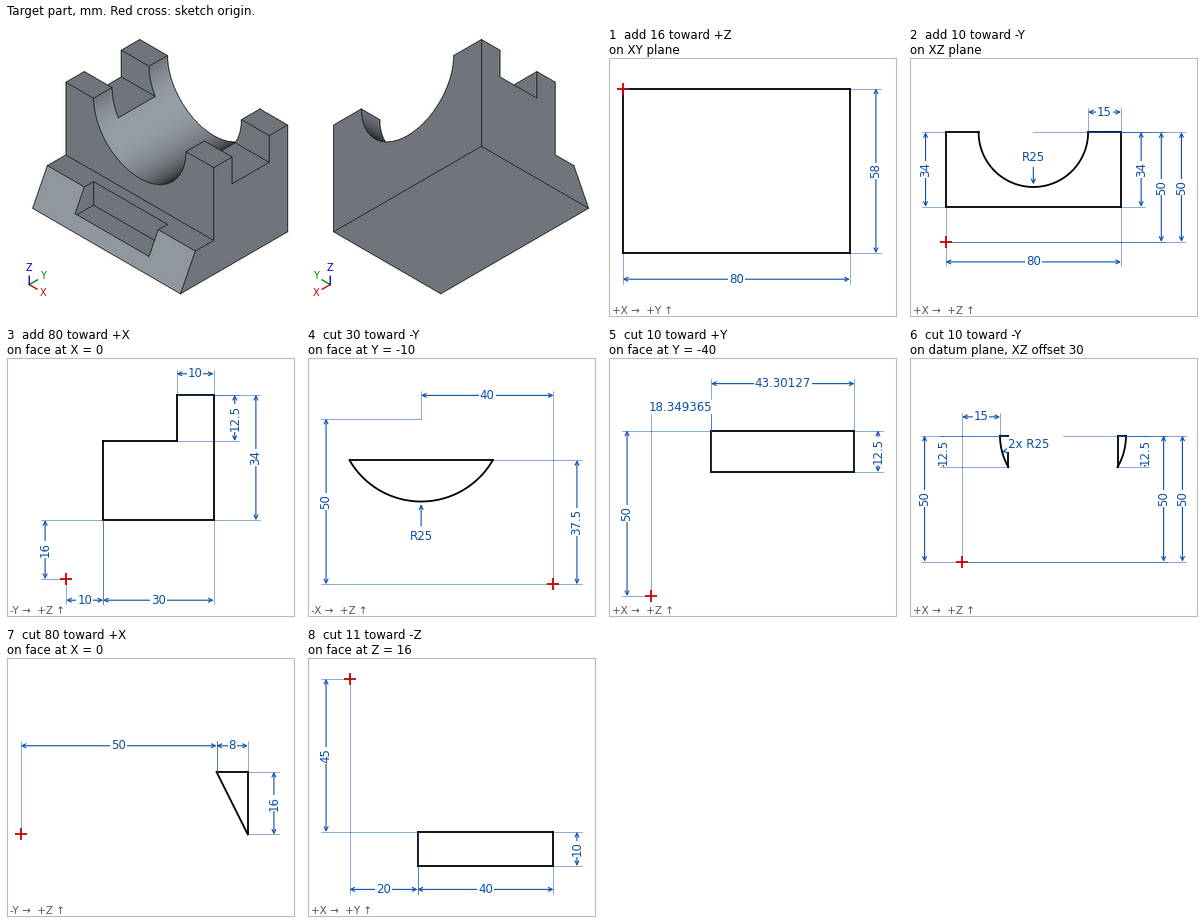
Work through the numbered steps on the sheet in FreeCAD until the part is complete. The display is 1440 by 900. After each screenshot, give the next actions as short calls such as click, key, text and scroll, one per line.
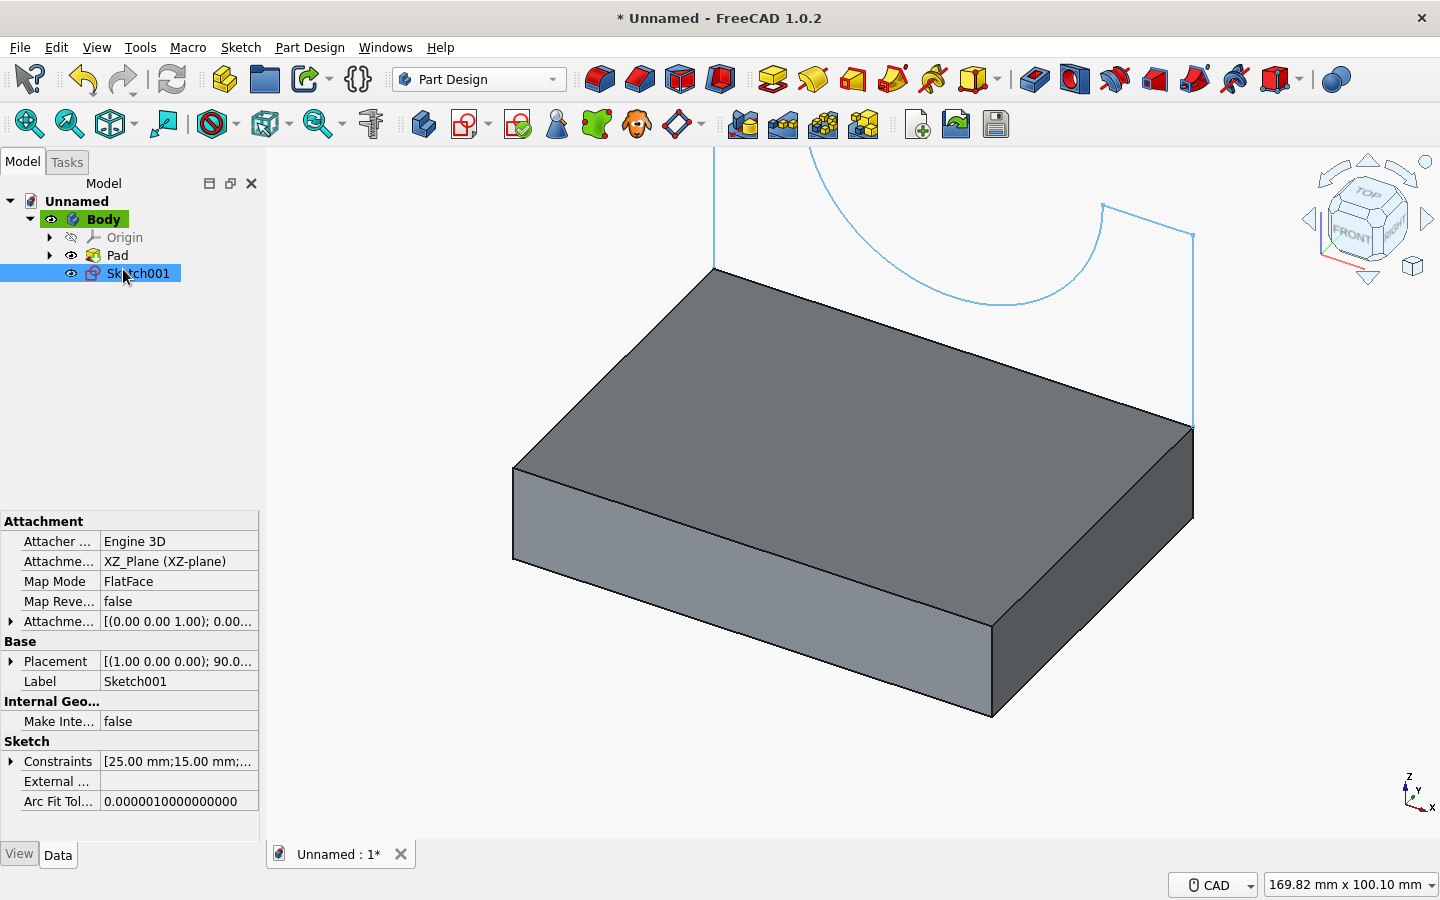
click(774, 80)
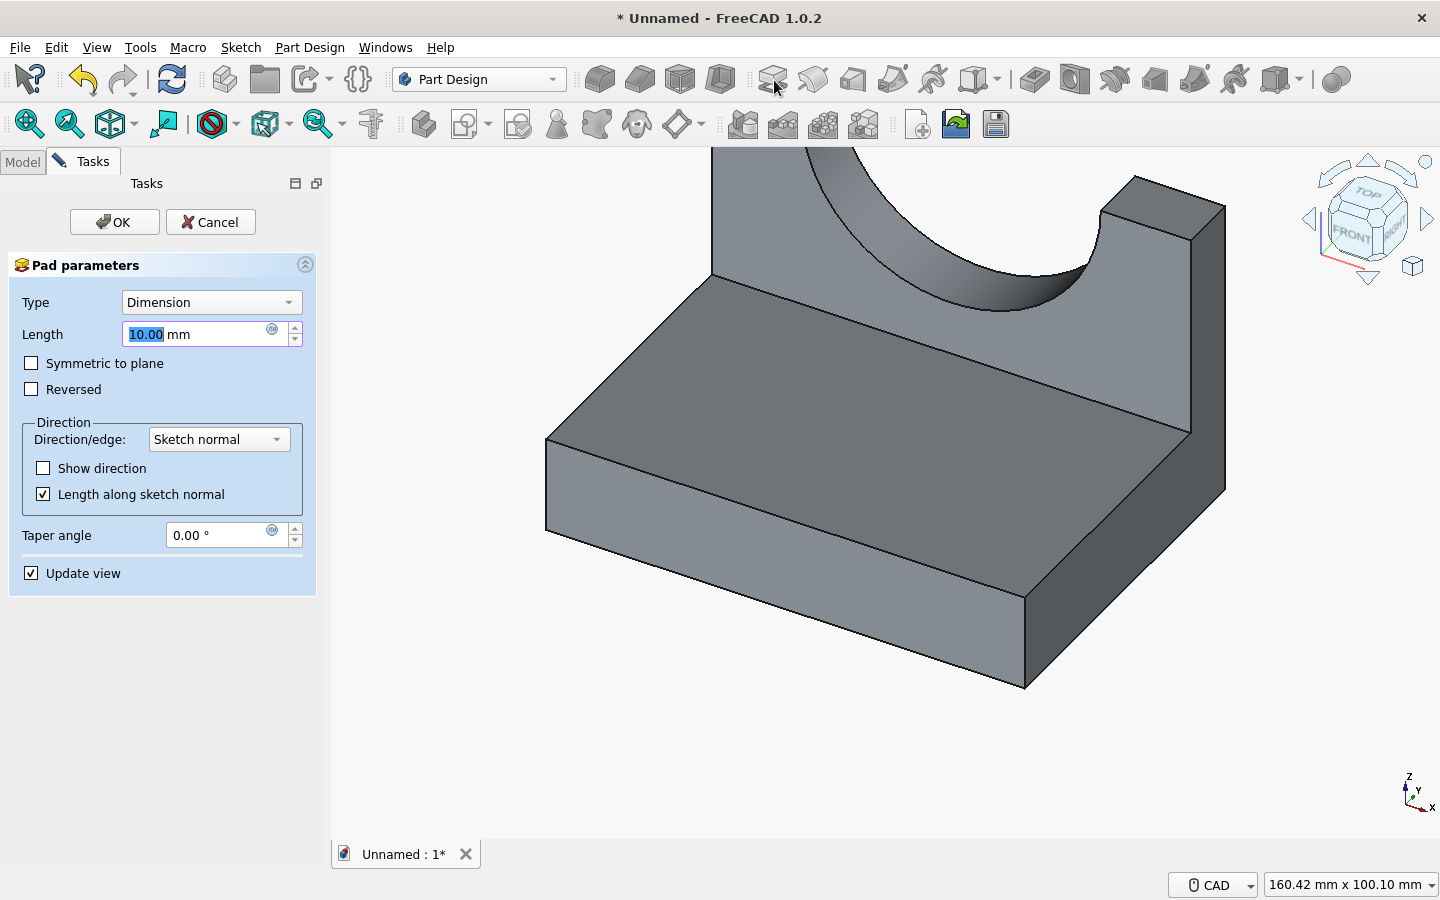
text(10)
key(Tab)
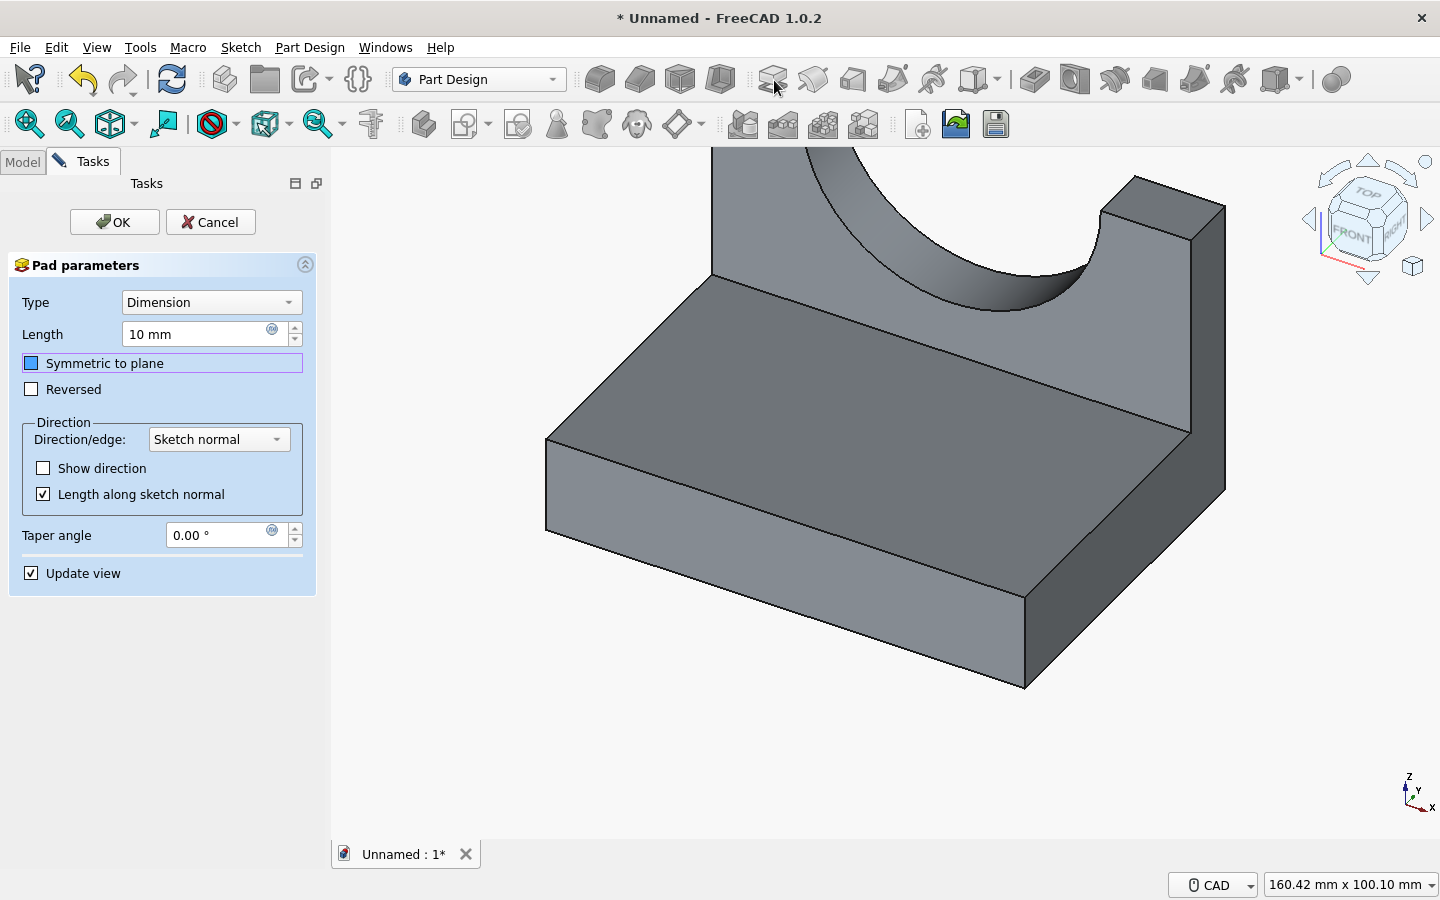
click(115, 222)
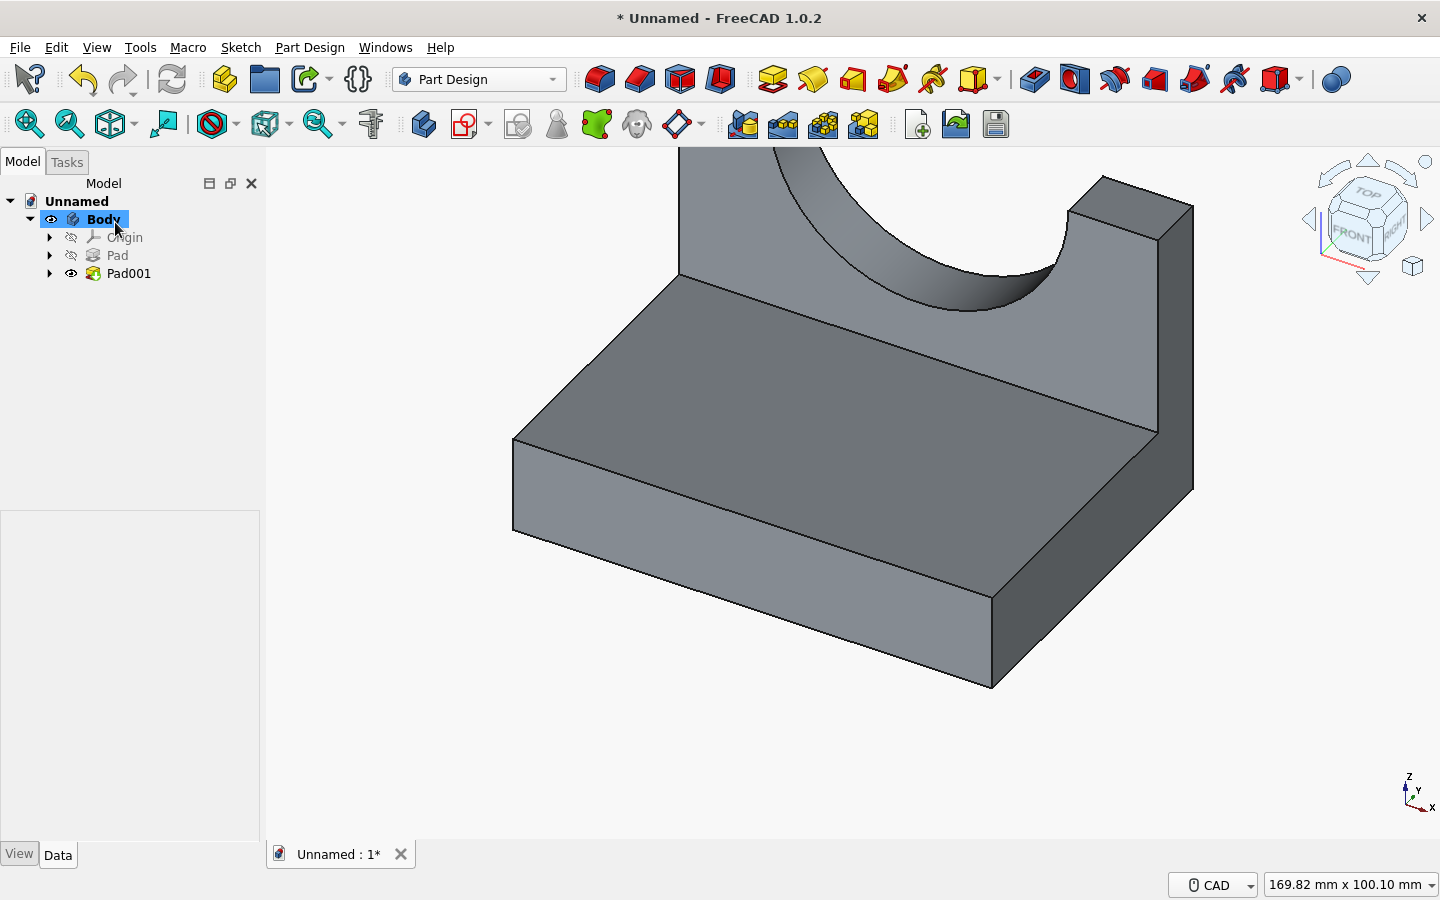
click(30, 124)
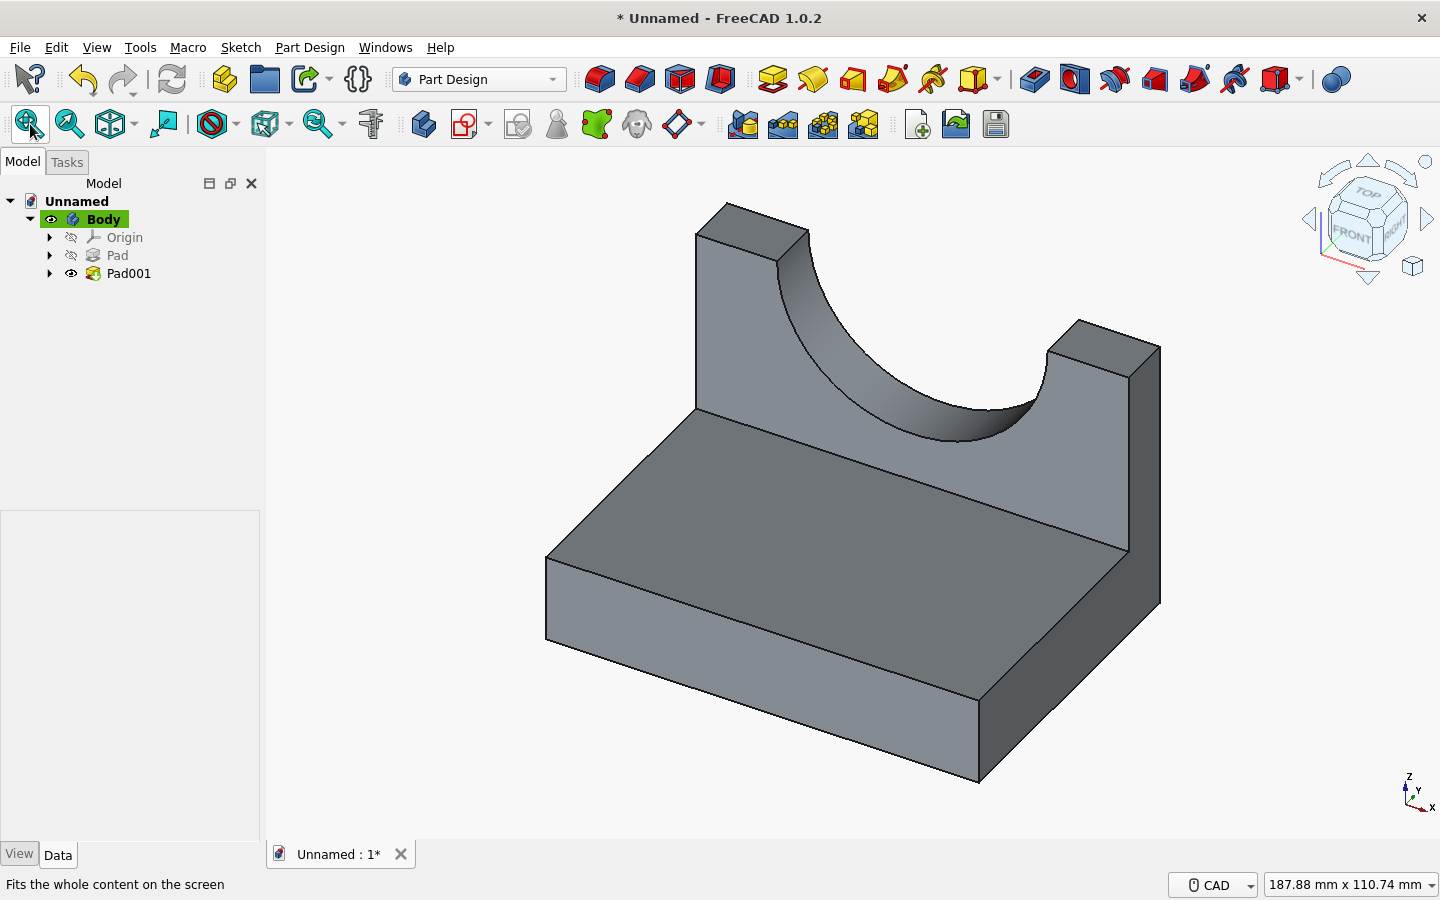
key(6)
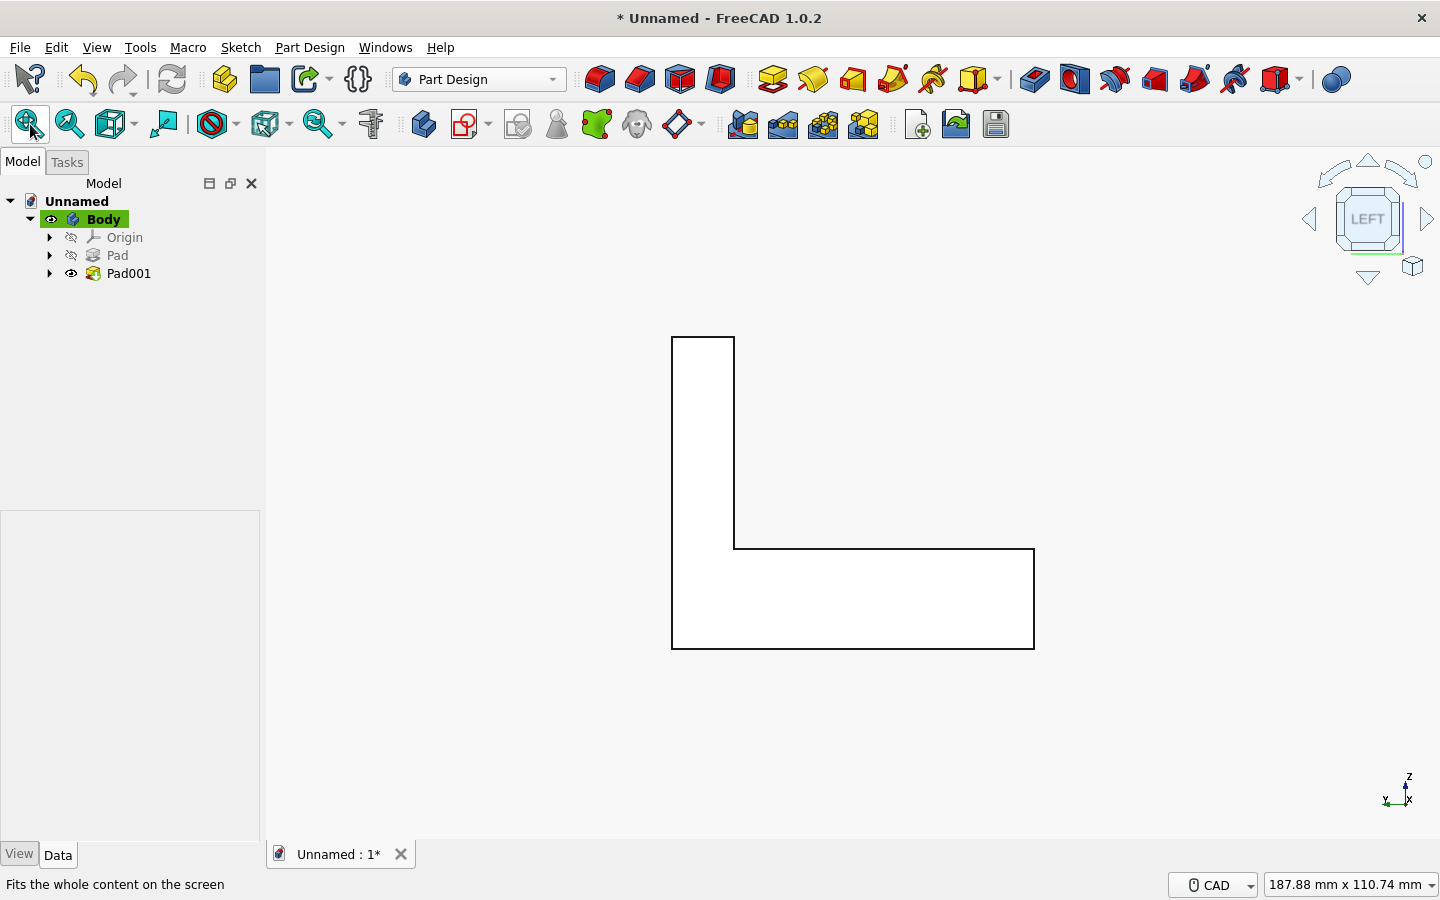
click(749, 581)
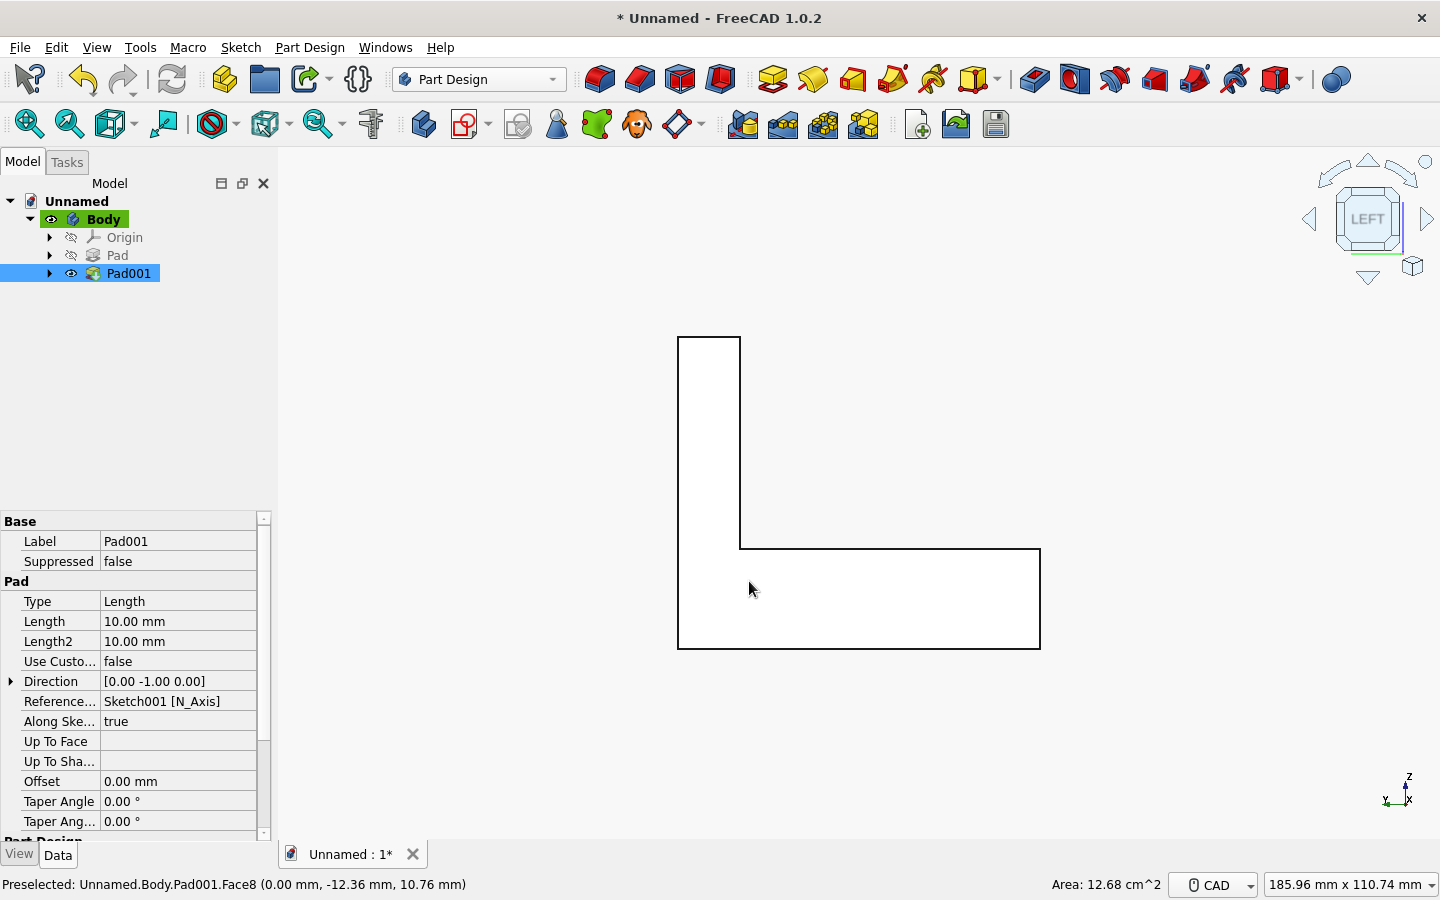
click(464, 124)